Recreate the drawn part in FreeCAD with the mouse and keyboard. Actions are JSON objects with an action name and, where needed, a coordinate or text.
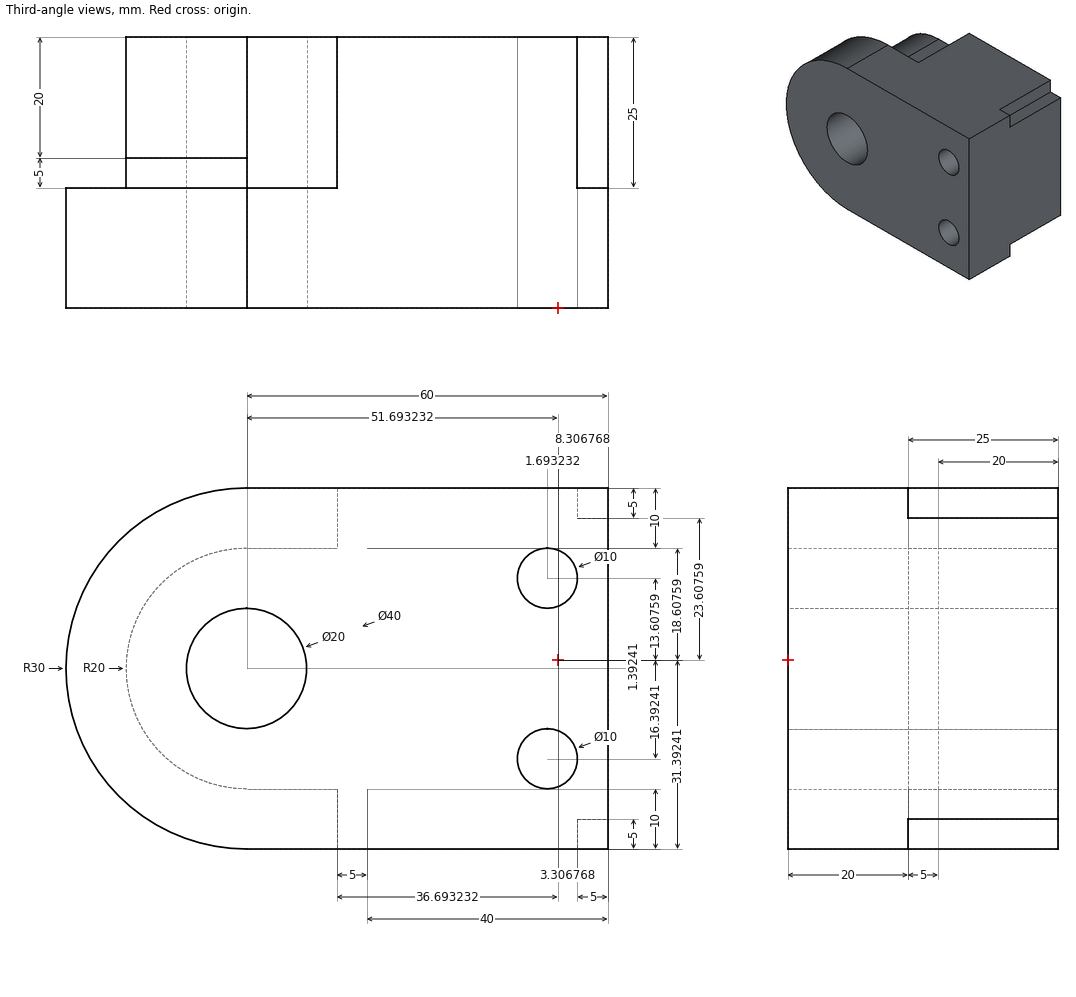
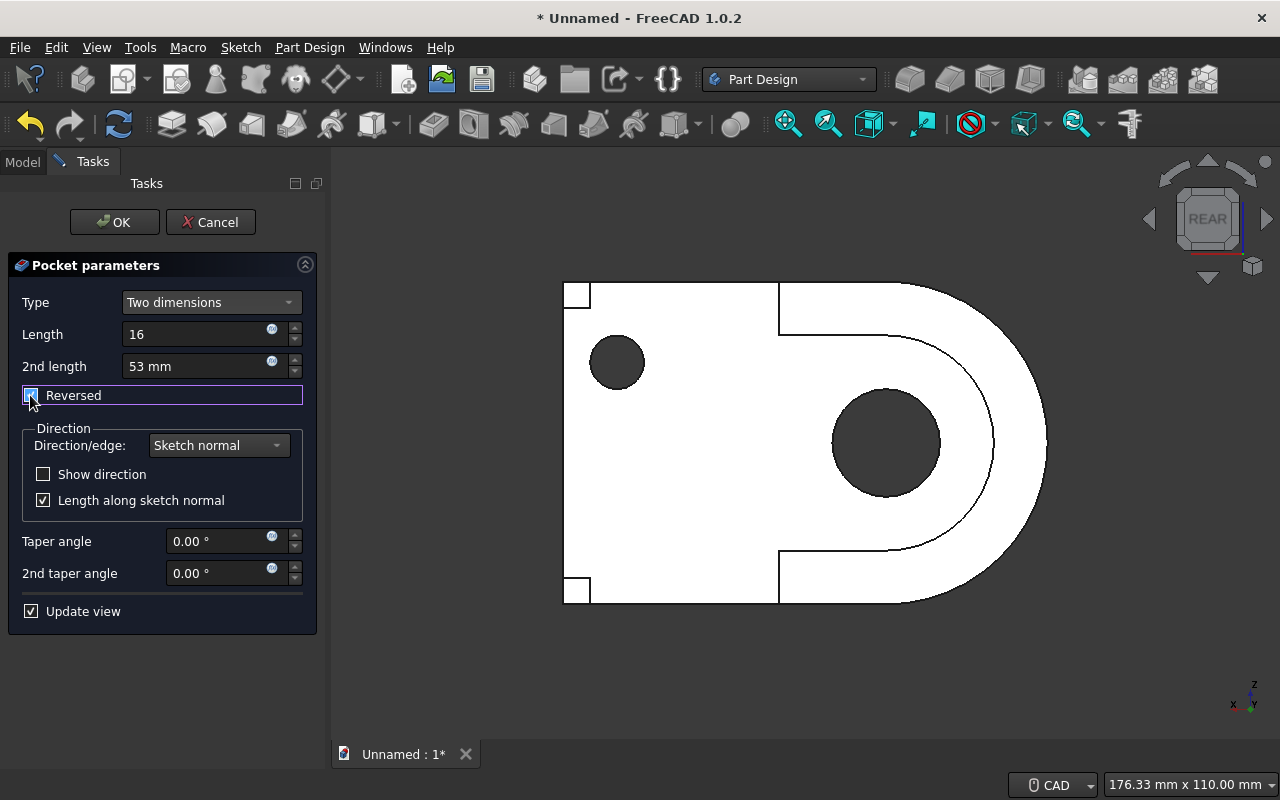
{"action": "left_click", "coordinate": [115, 222]}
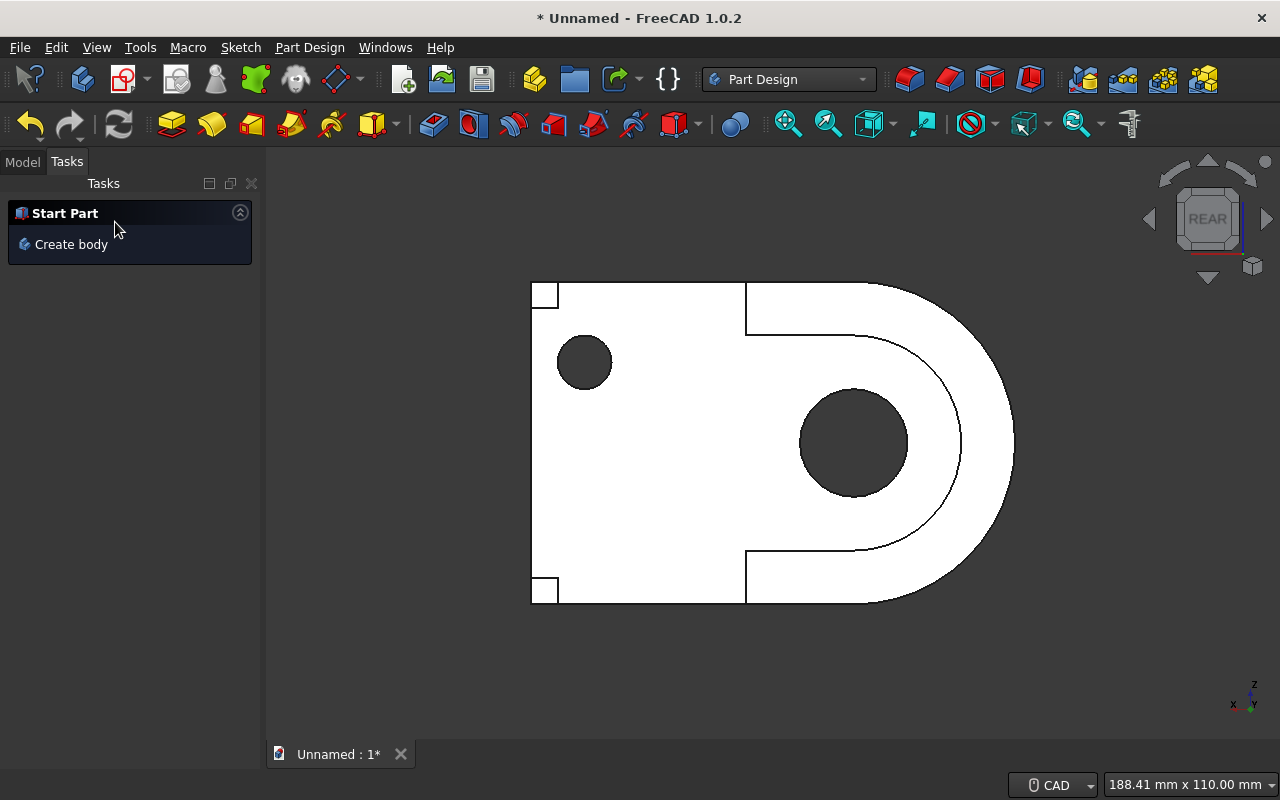
{"action": "left_click", "coordinate": [685, 442]}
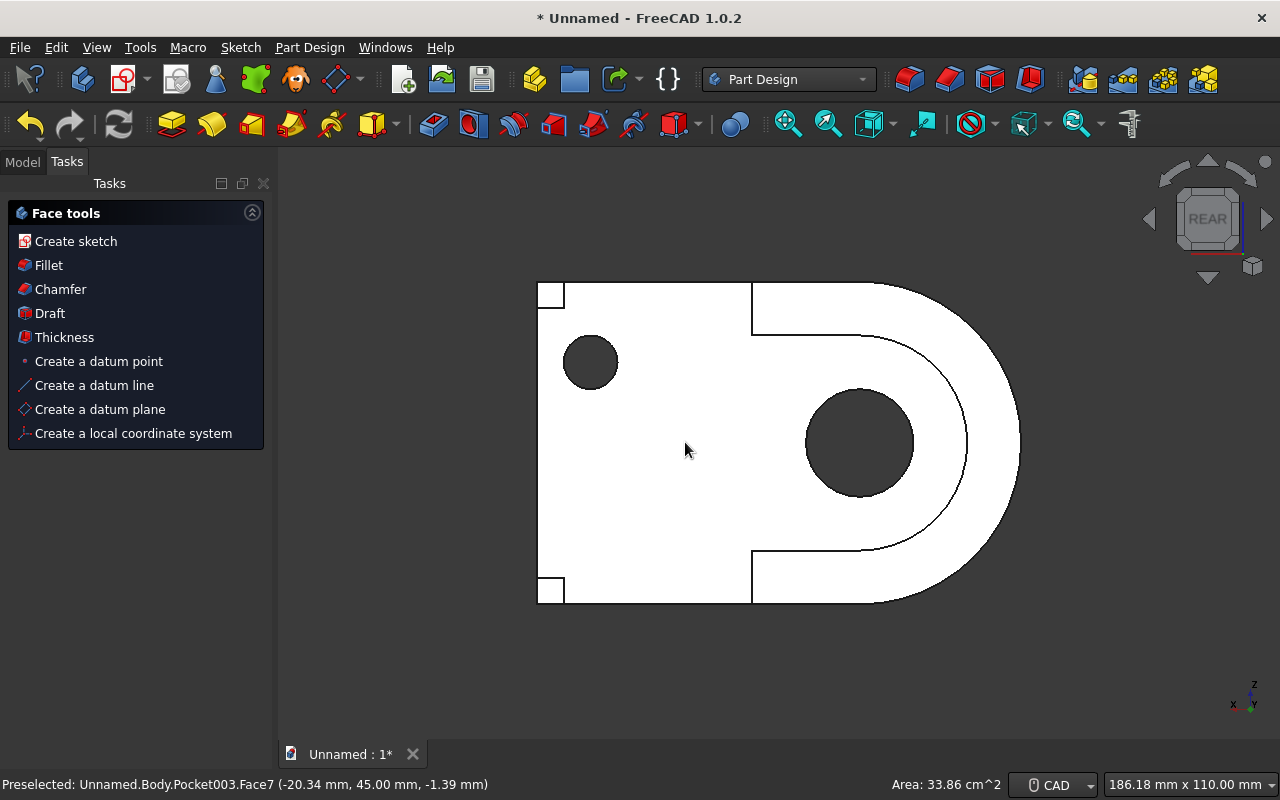
{"action": "left_click", "coordinate": [124, 80]}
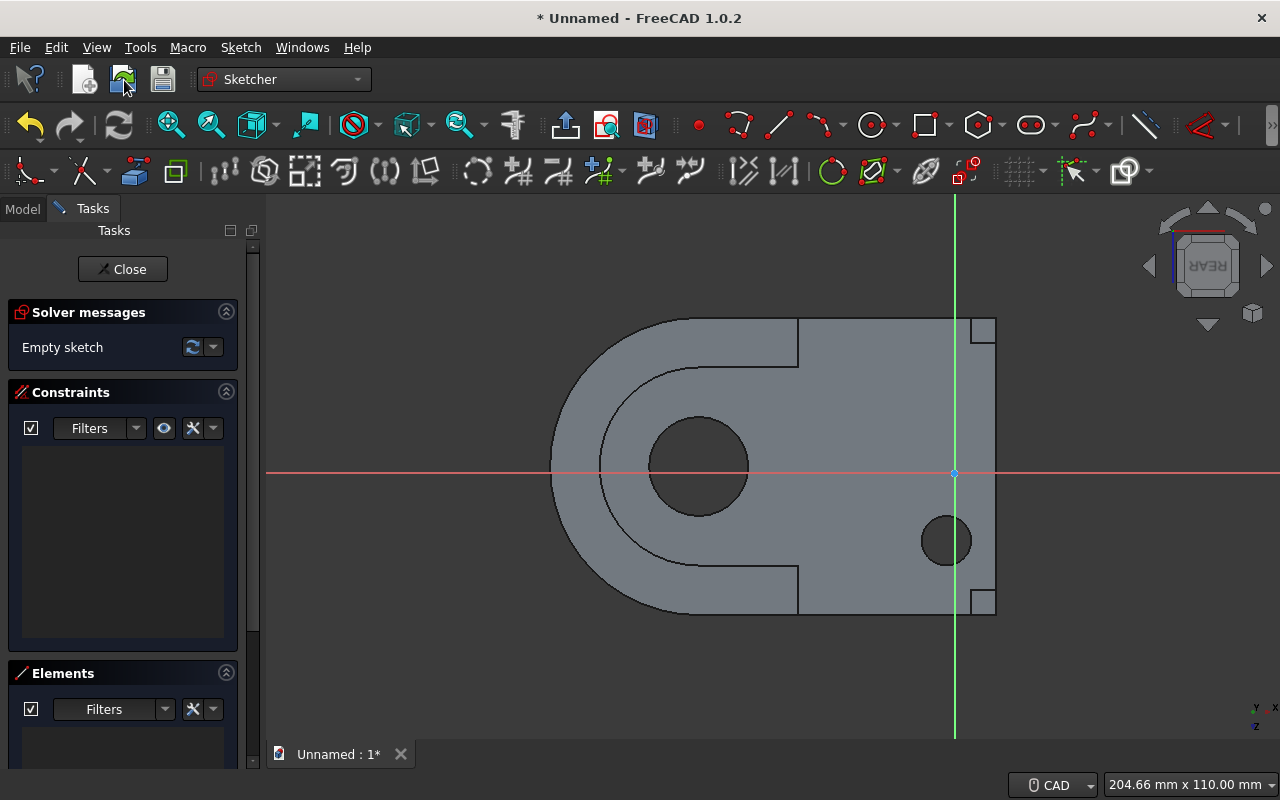
{"action": "scroll", "coordinate": [1051, 401], "scroll_direction": "up", "scroll_amount": 6}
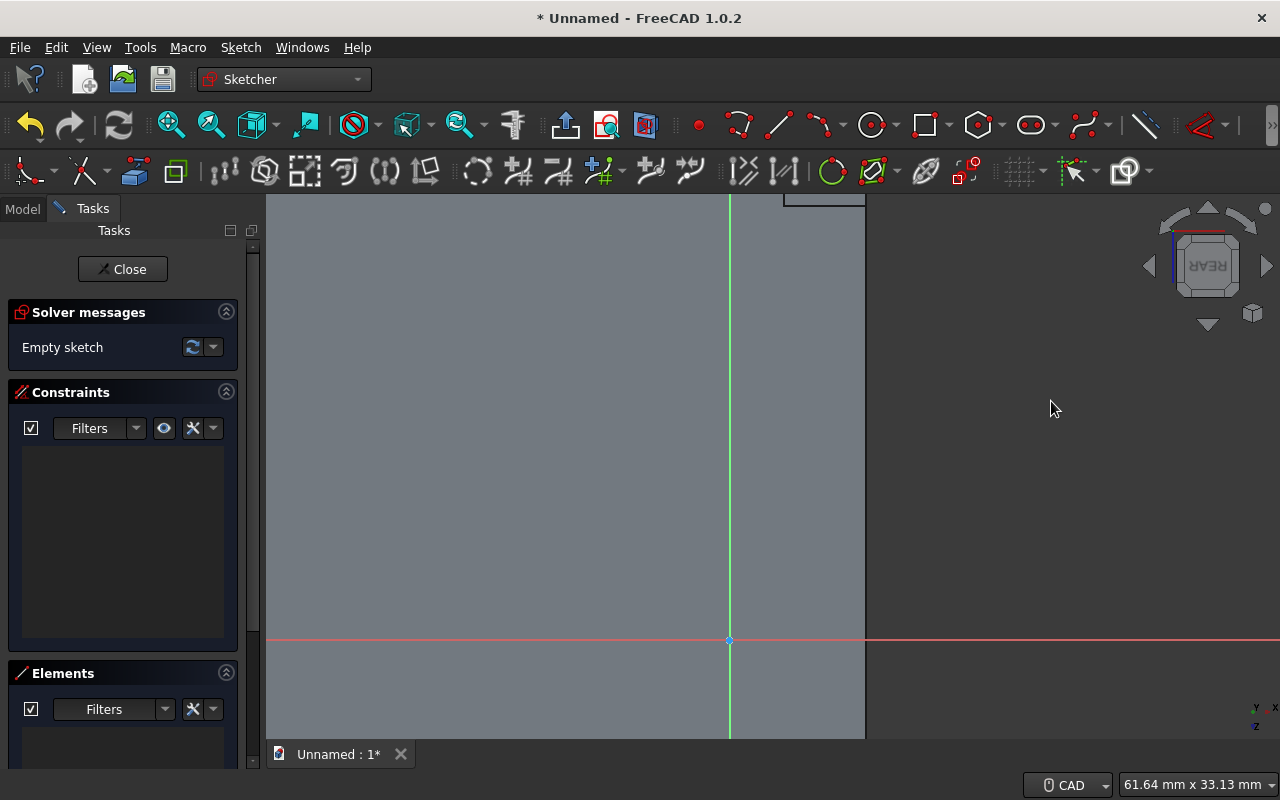
{"action": "key", "text": "g c"}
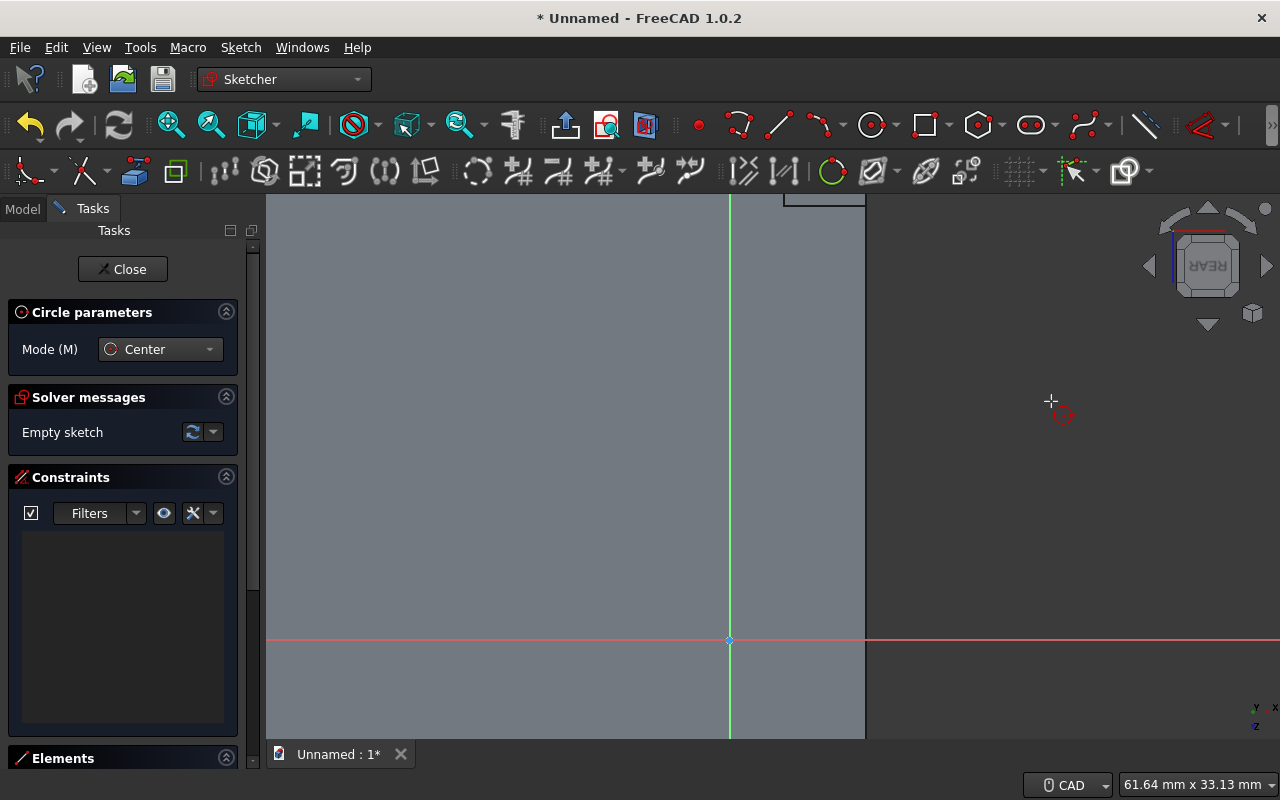
{"action": "left_click", "coordinate": [702, 371]}
{"action": "left_click", "coordinate": [760, 313]}
{"action": "key", "text": "Escape"}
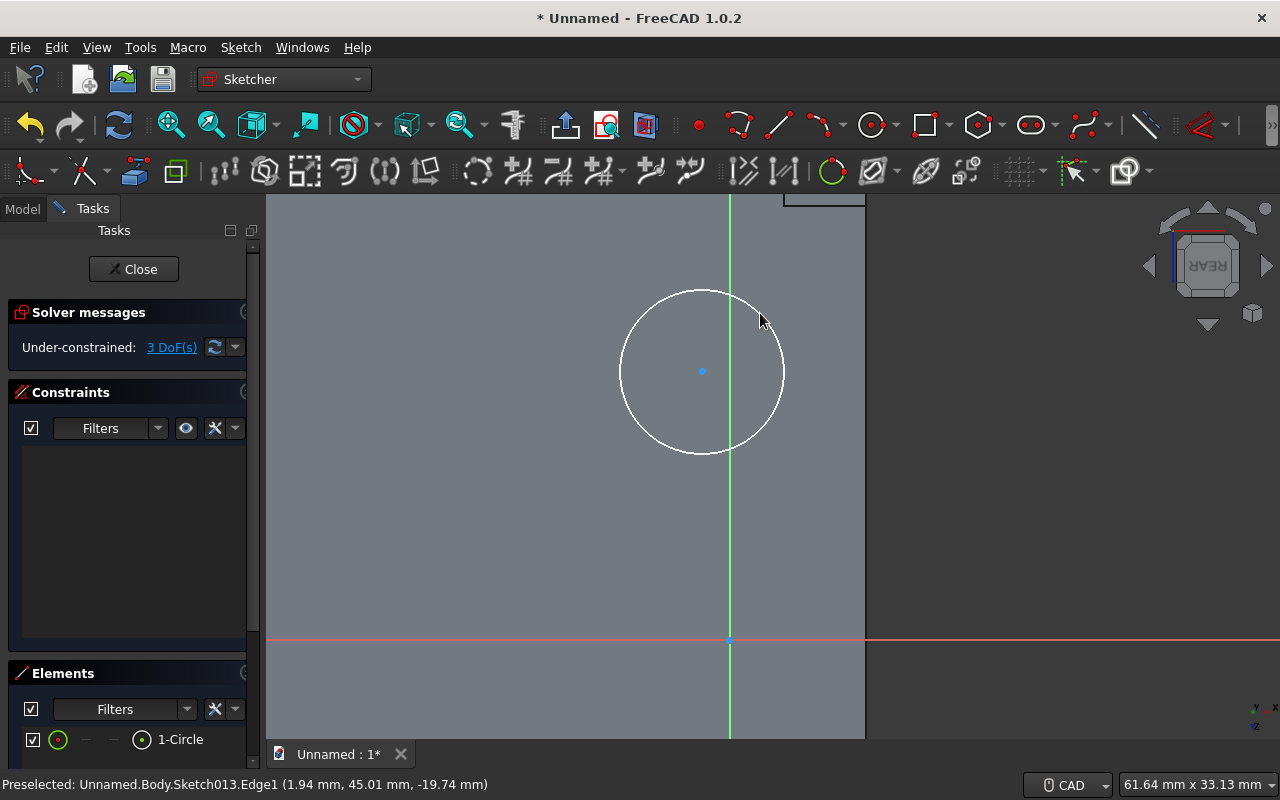
{"action": "key", "text": "d"}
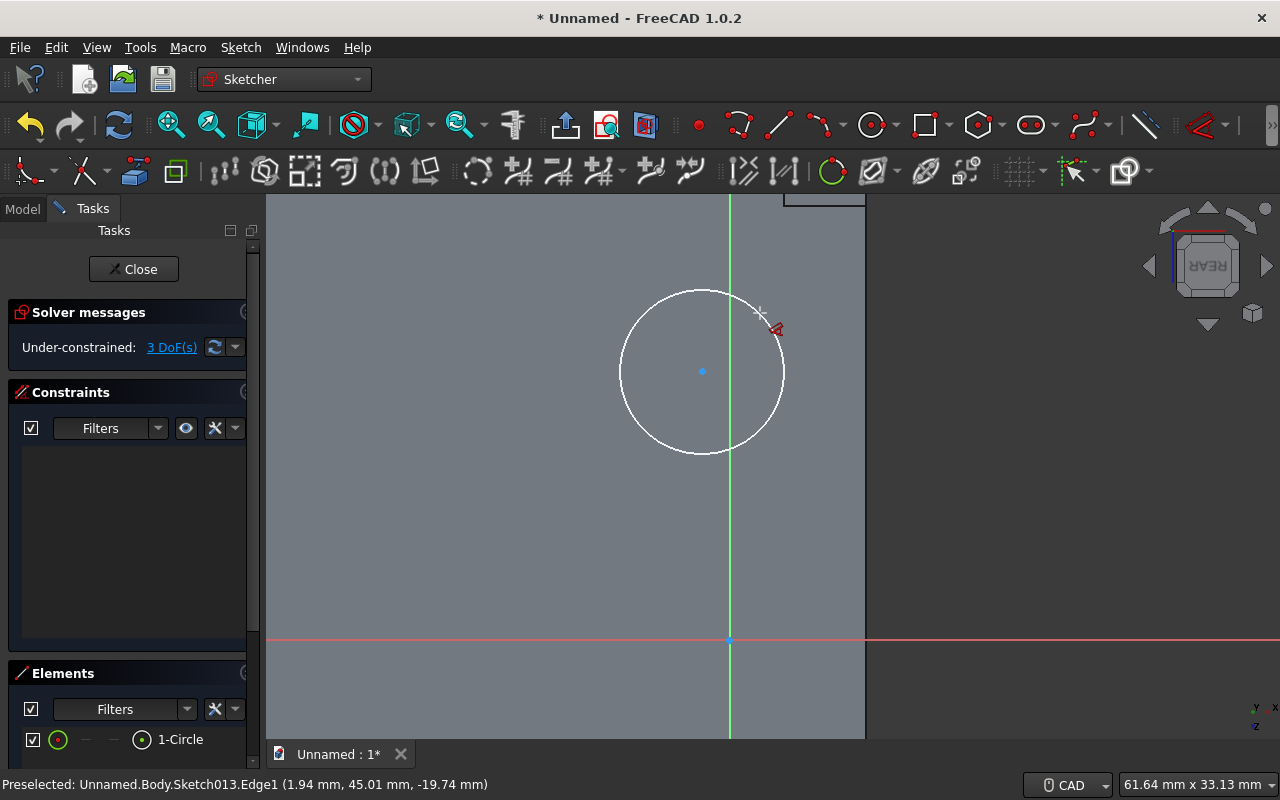
{"action": "left_click", "coordinate": [760, 314]}
{"action": "left_click", "coordinate": [783, 291]}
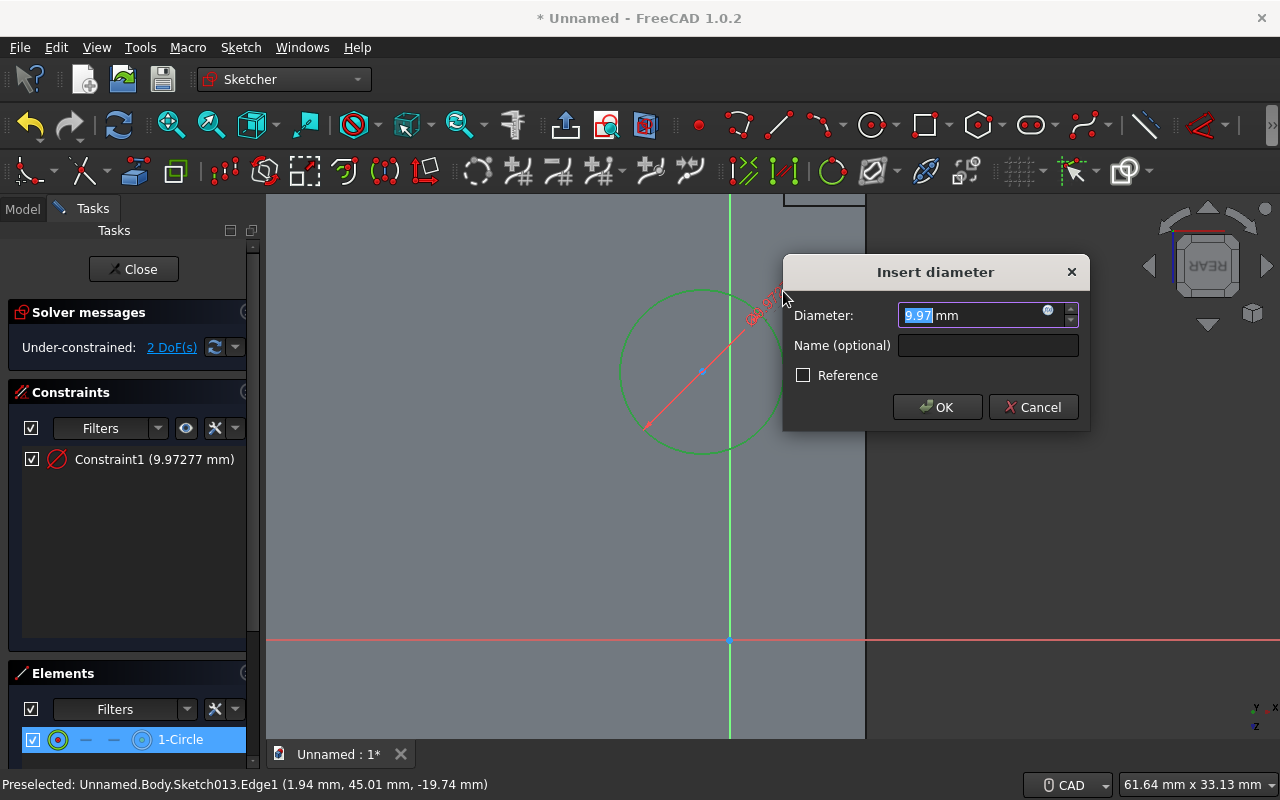
{"action": "type", "text": "10"}
{"action": "key", "text": "Return"}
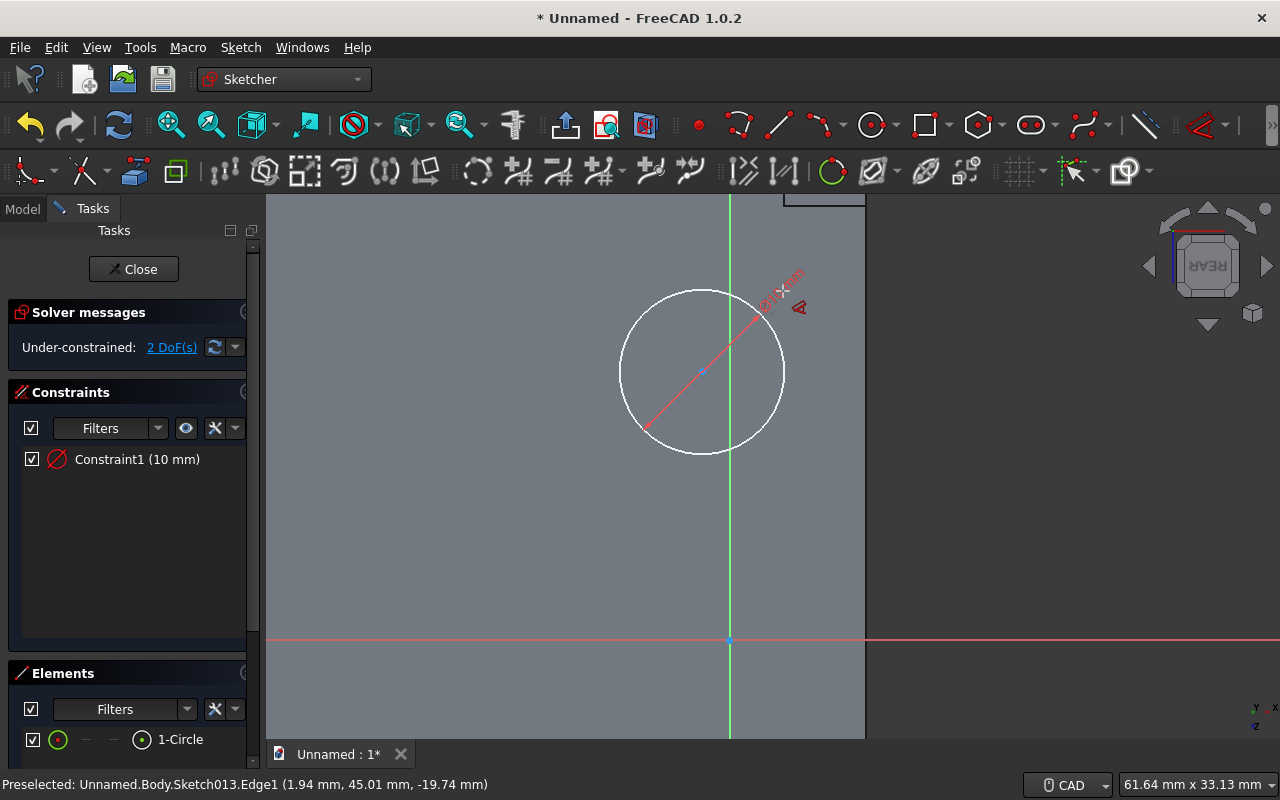
{"action": "scroll", "coordinate": [702, 372], "scroll_direction": "up", "scroll_amount": 2}